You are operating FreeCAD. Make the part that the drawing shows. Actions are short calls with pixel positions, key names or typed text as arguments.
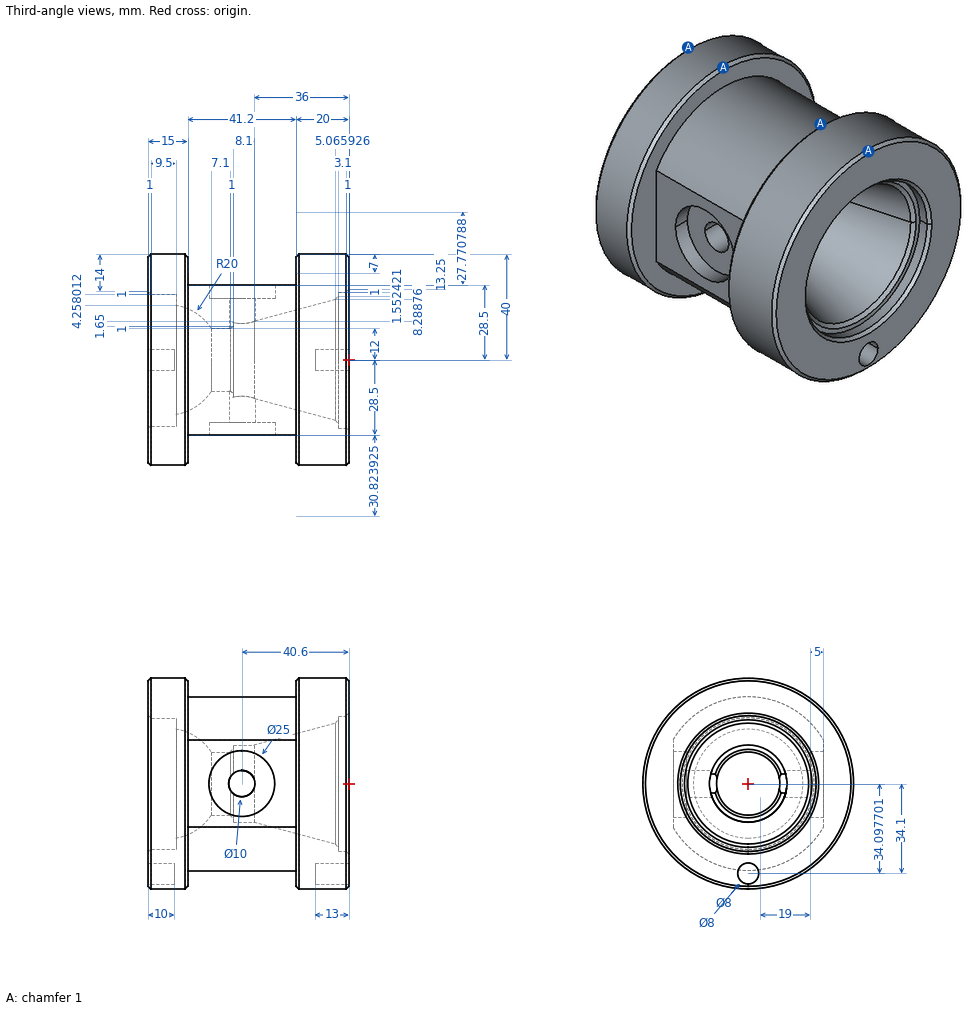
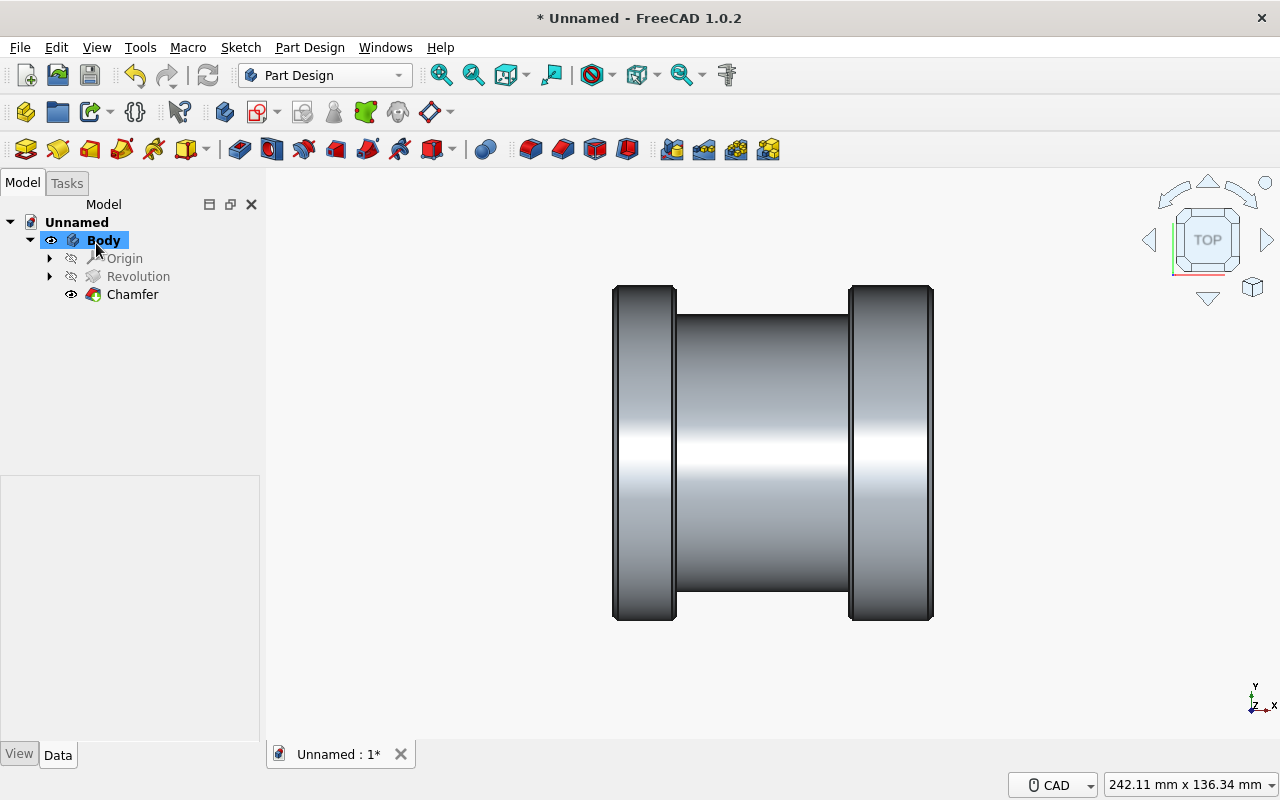
click(258, 112)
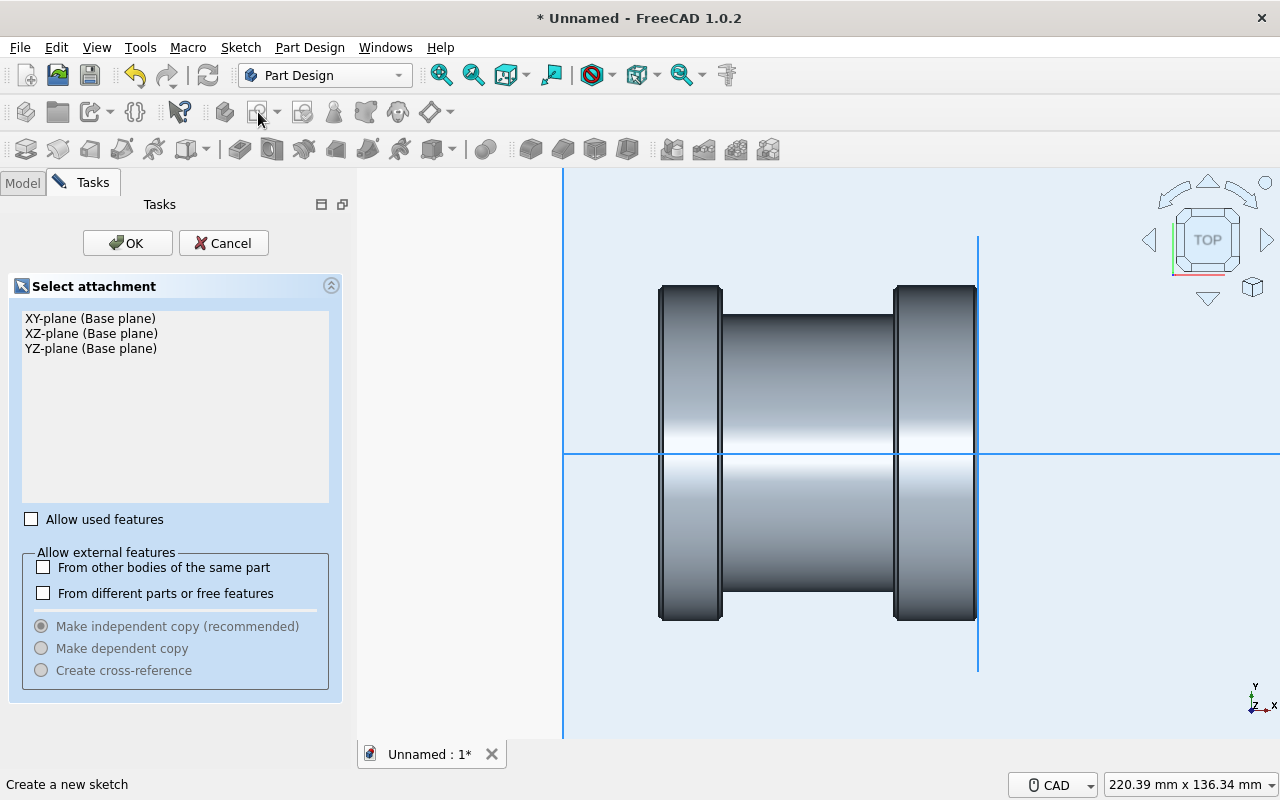
click(82, 318)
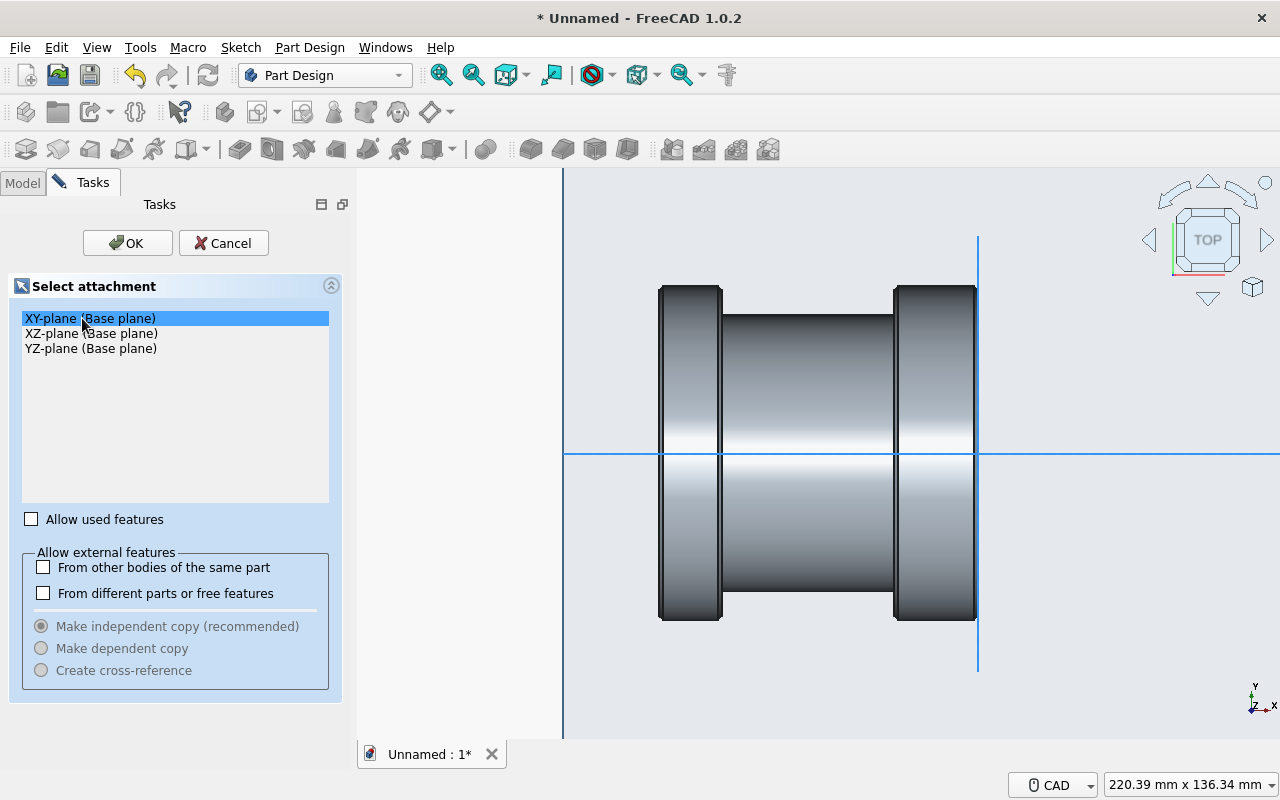
click(128, 243)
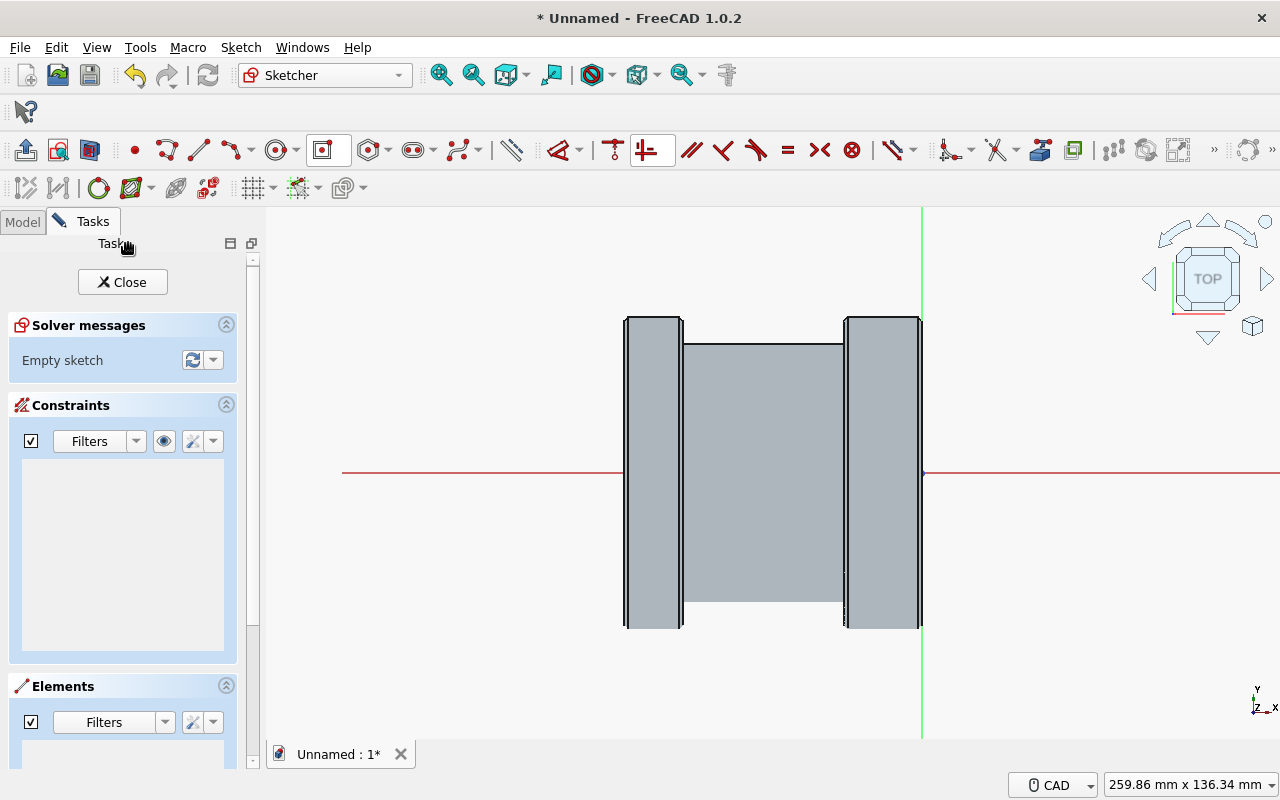
click(90, 150)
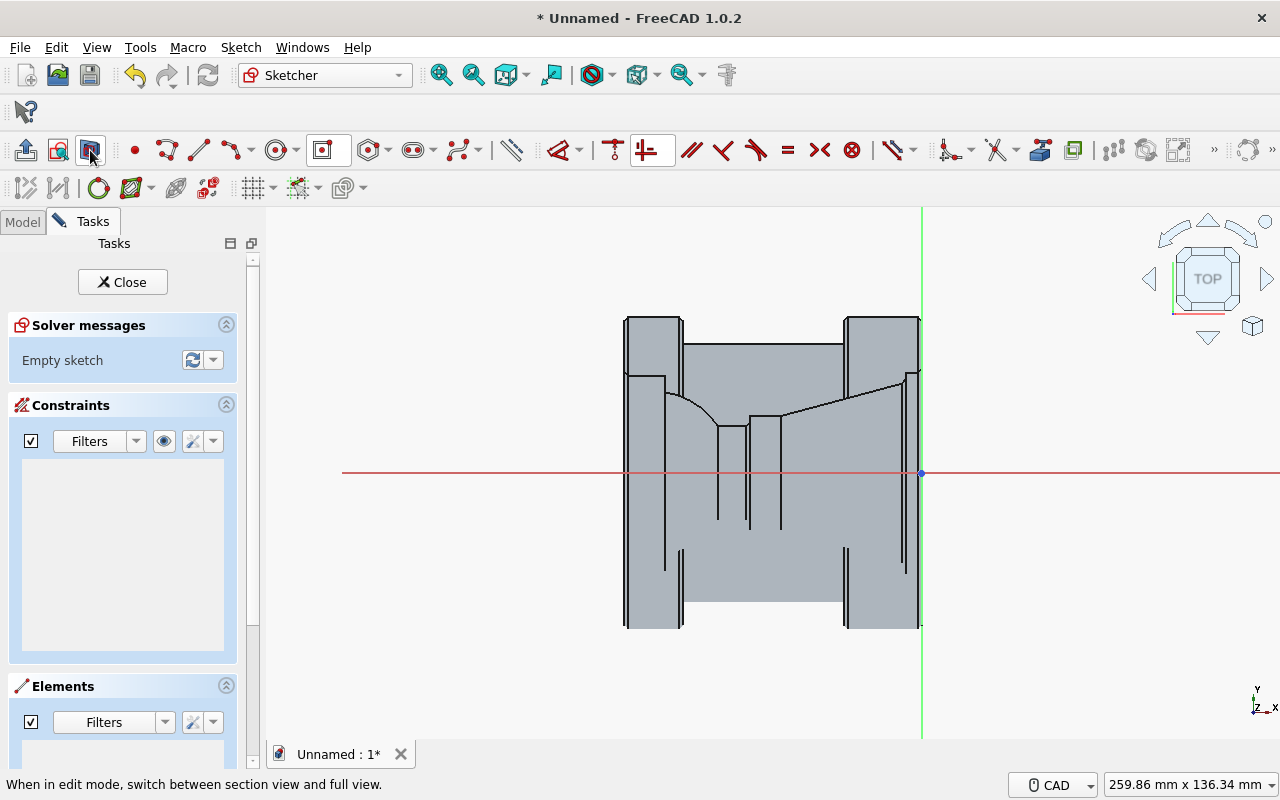
scroll(294, 445, down, 1)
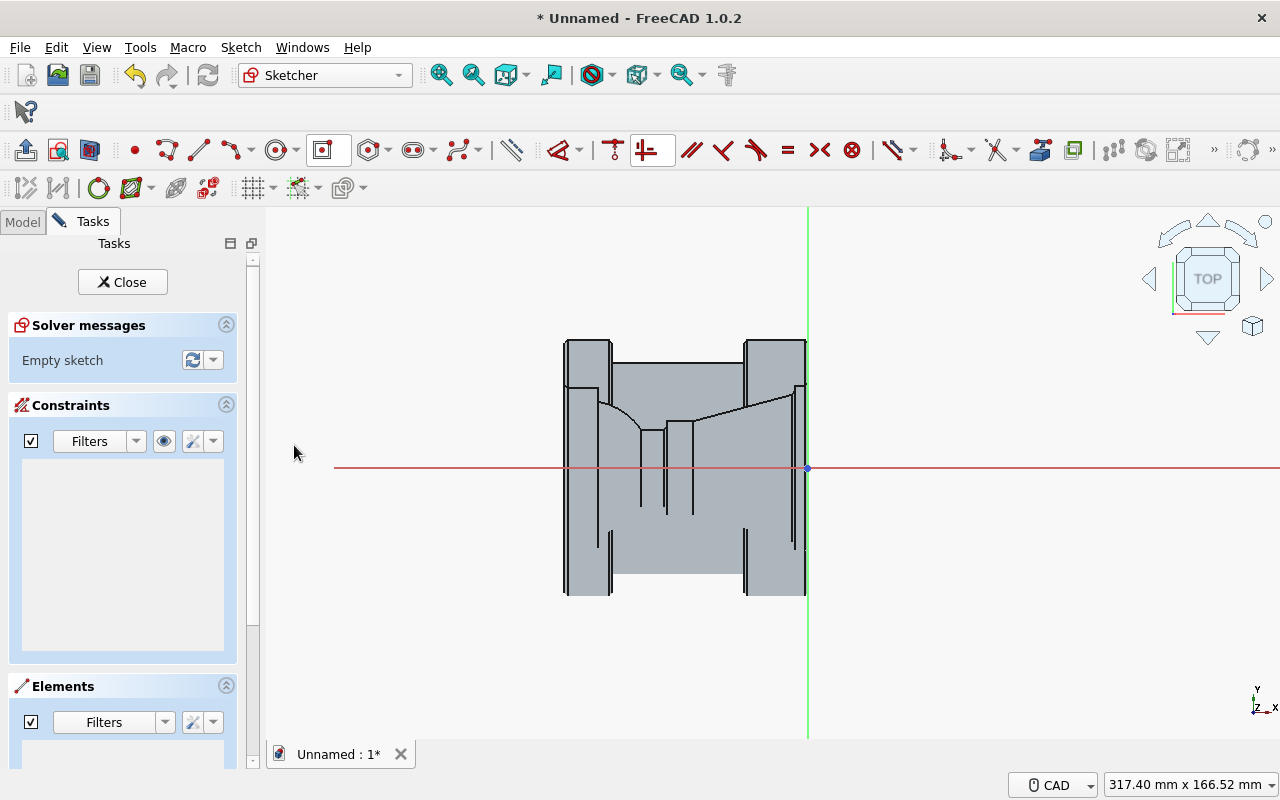
key(g)
key(r)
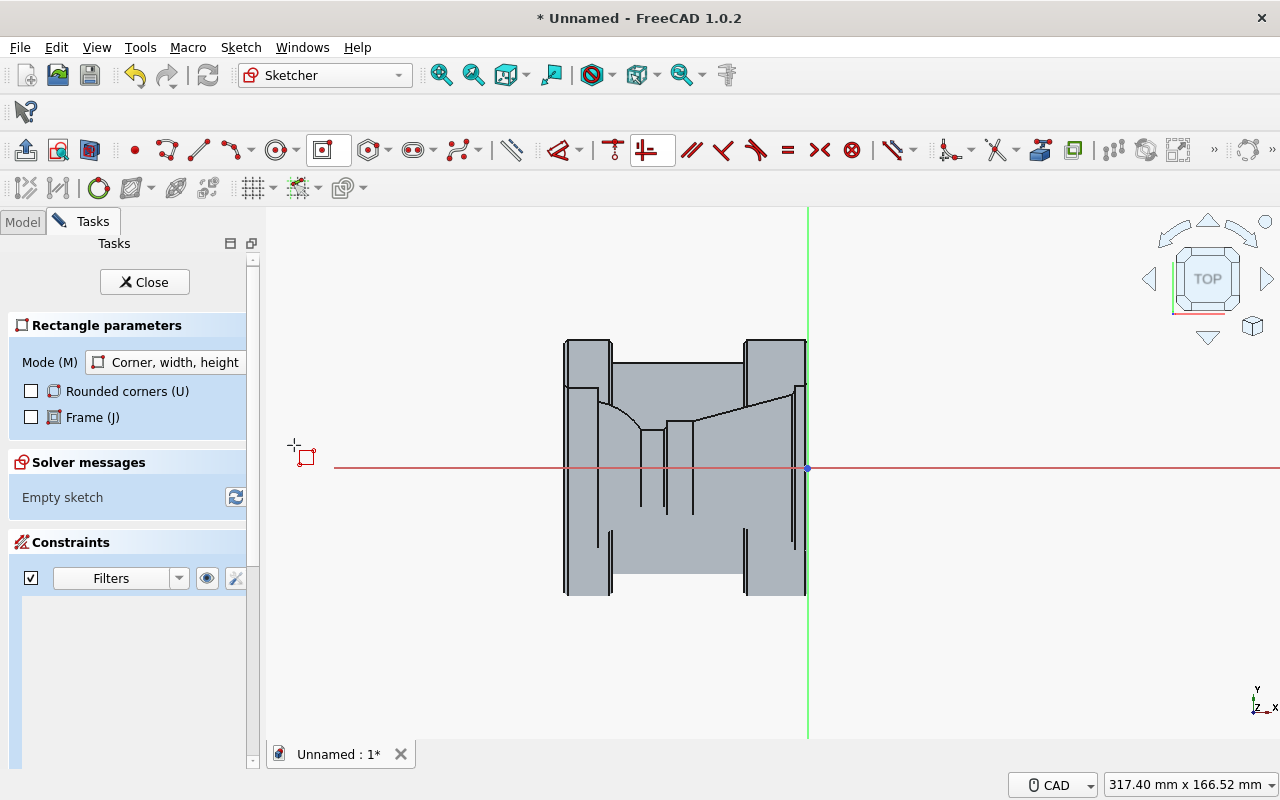
click(612, 288)
move(744, 377)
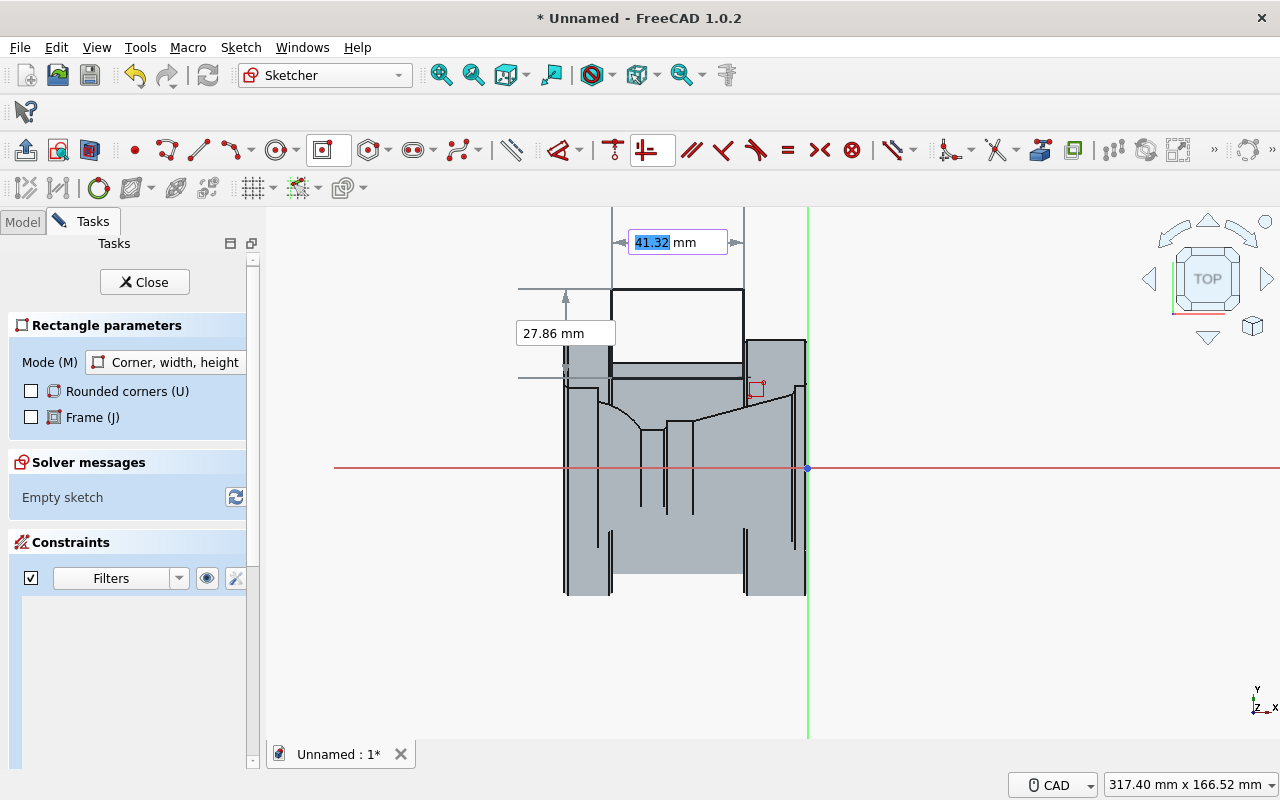
text(41.2)
key(Tab)
text(27.770788)
key(Return)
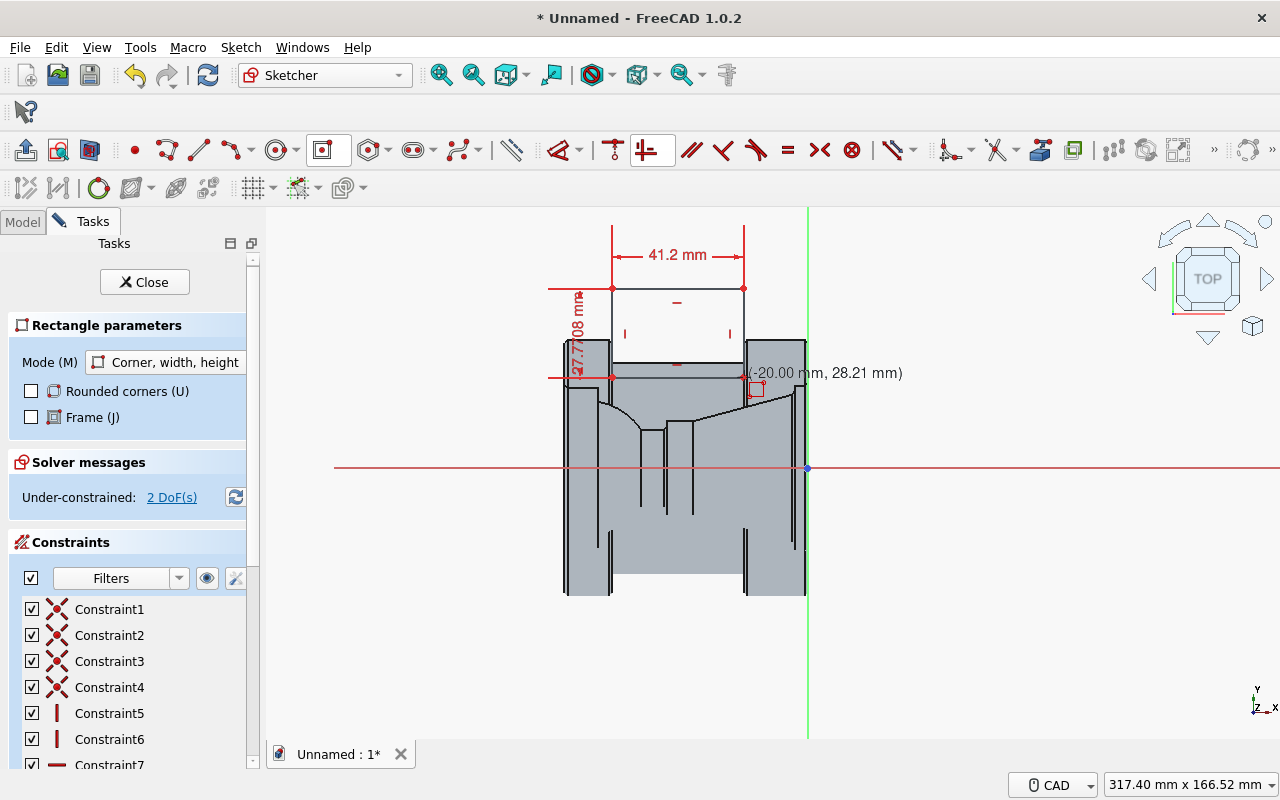
click(612, 559)
move(744, 658)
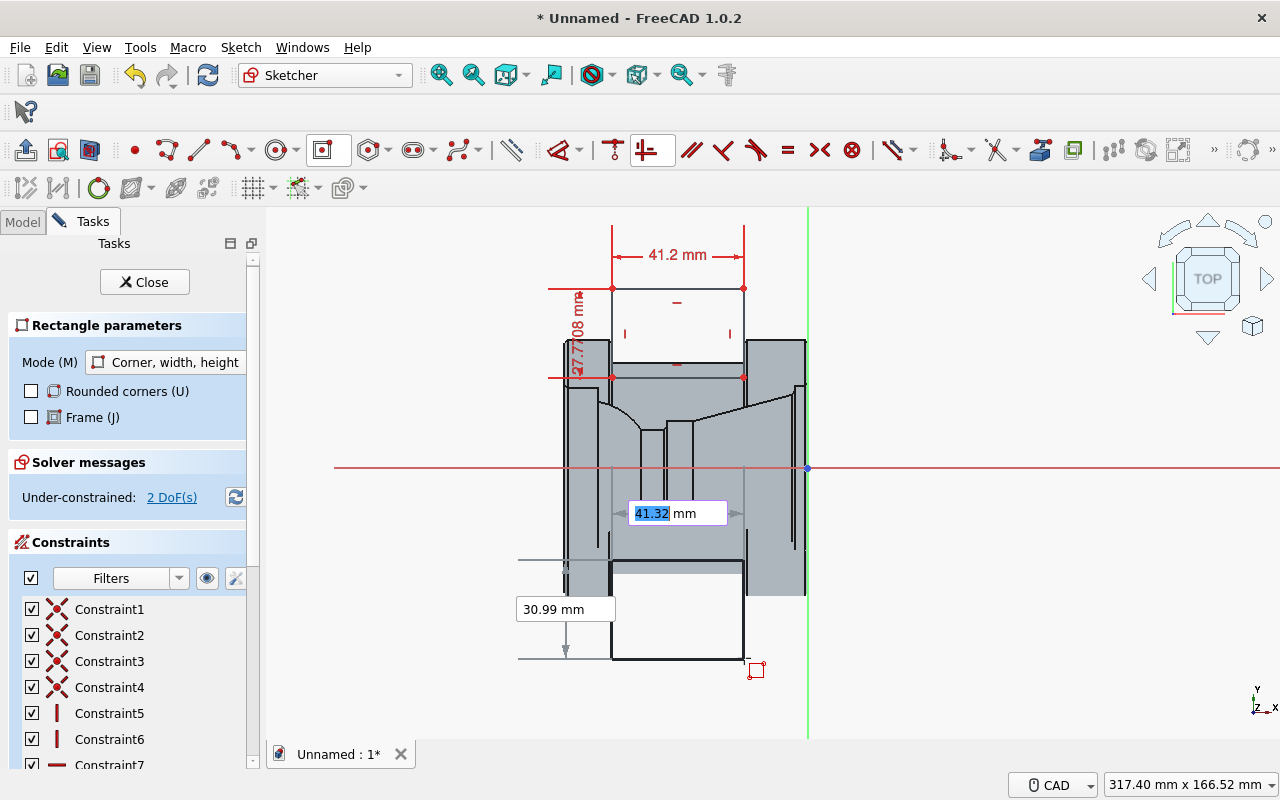
text(41.2)
key(Tab)
text(30.823925)
key(Return)
key(Escape)